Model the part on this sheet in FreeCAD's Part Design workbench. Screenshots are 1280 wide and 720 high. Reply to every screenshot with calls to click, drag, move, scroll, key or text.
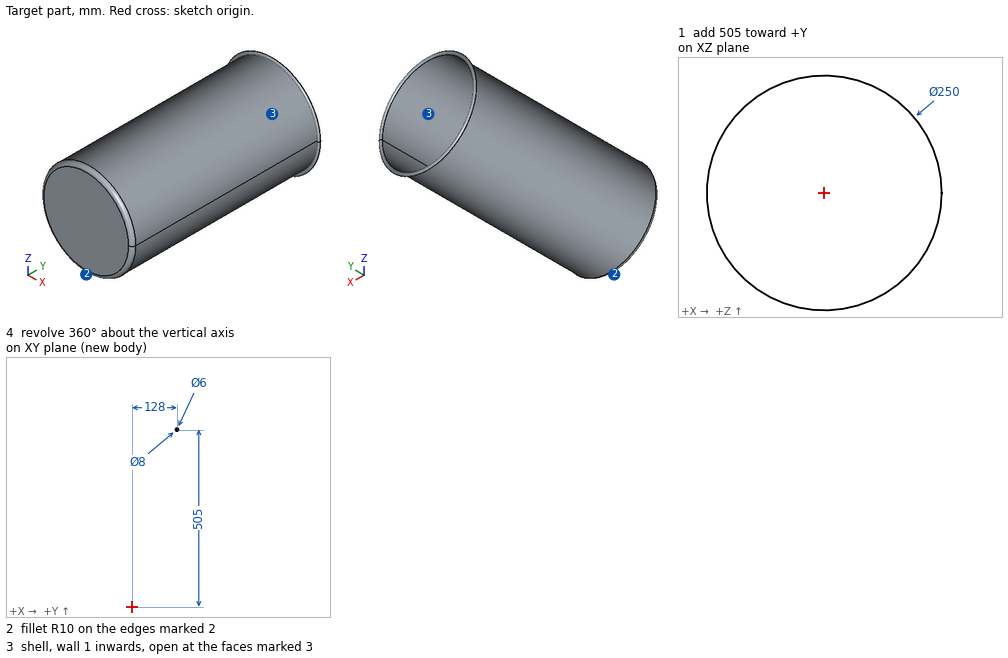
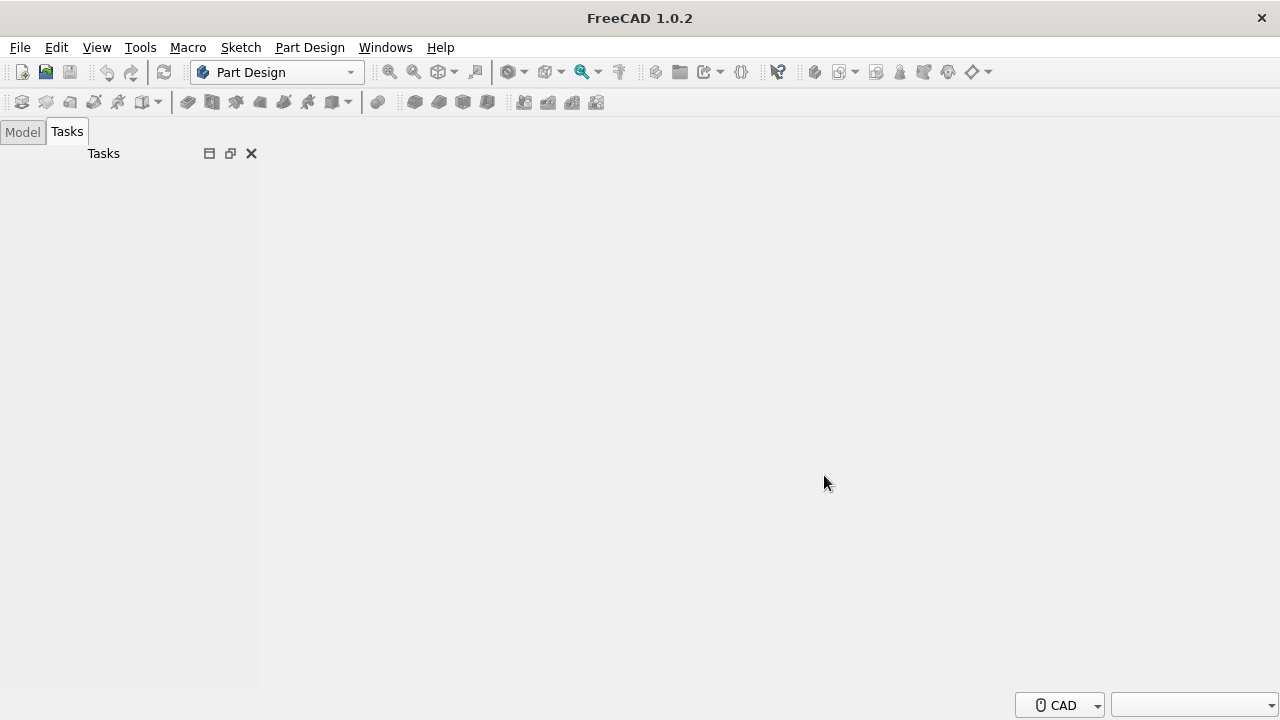
click(22, 72)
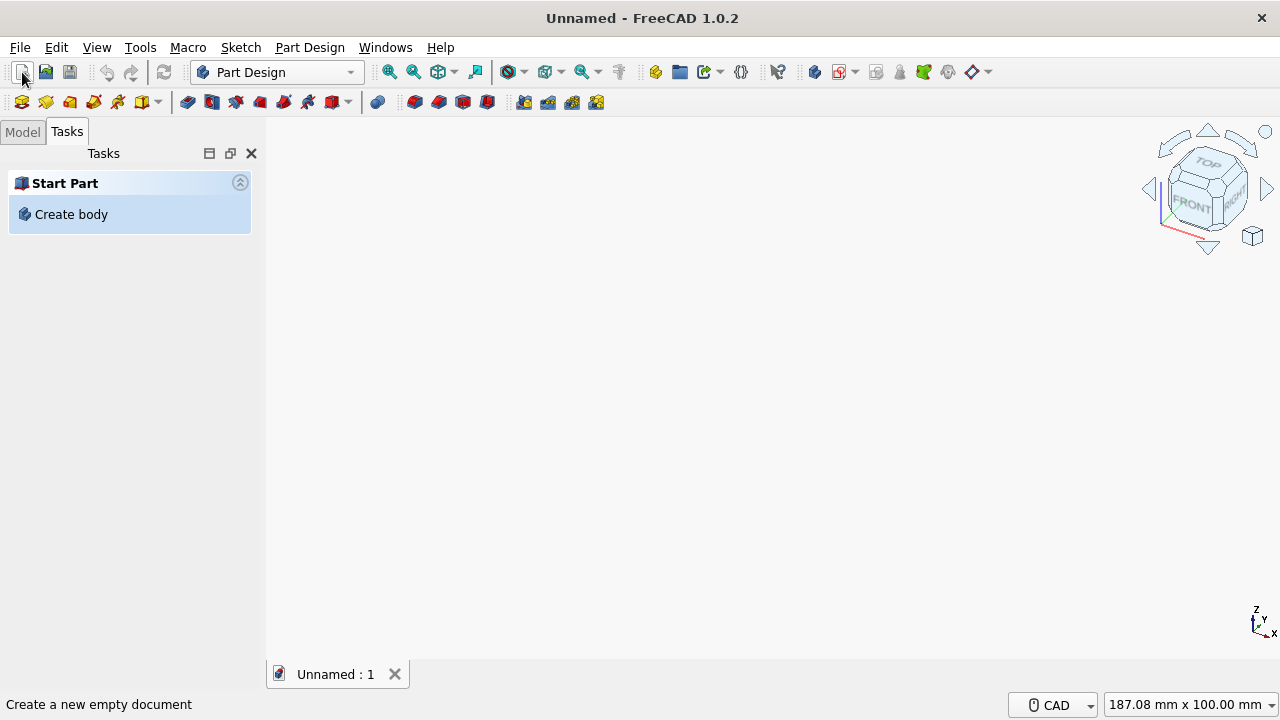
click(840, 72)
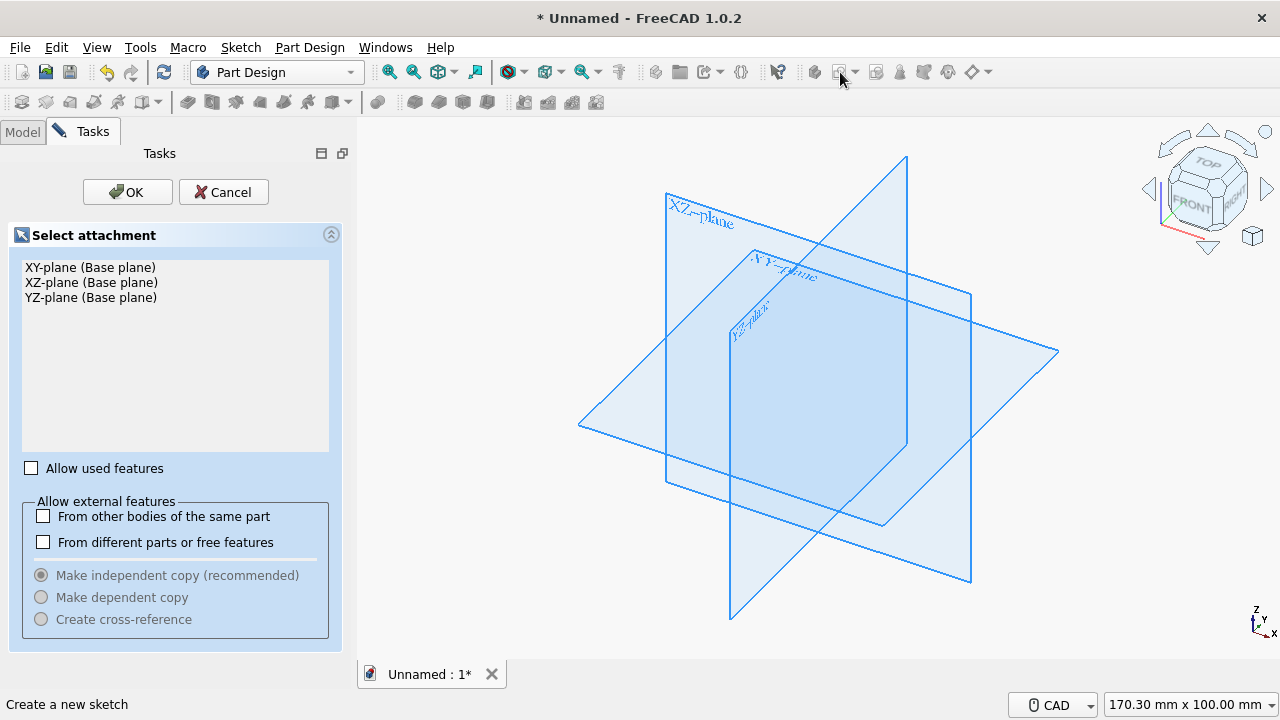
click(82, 282)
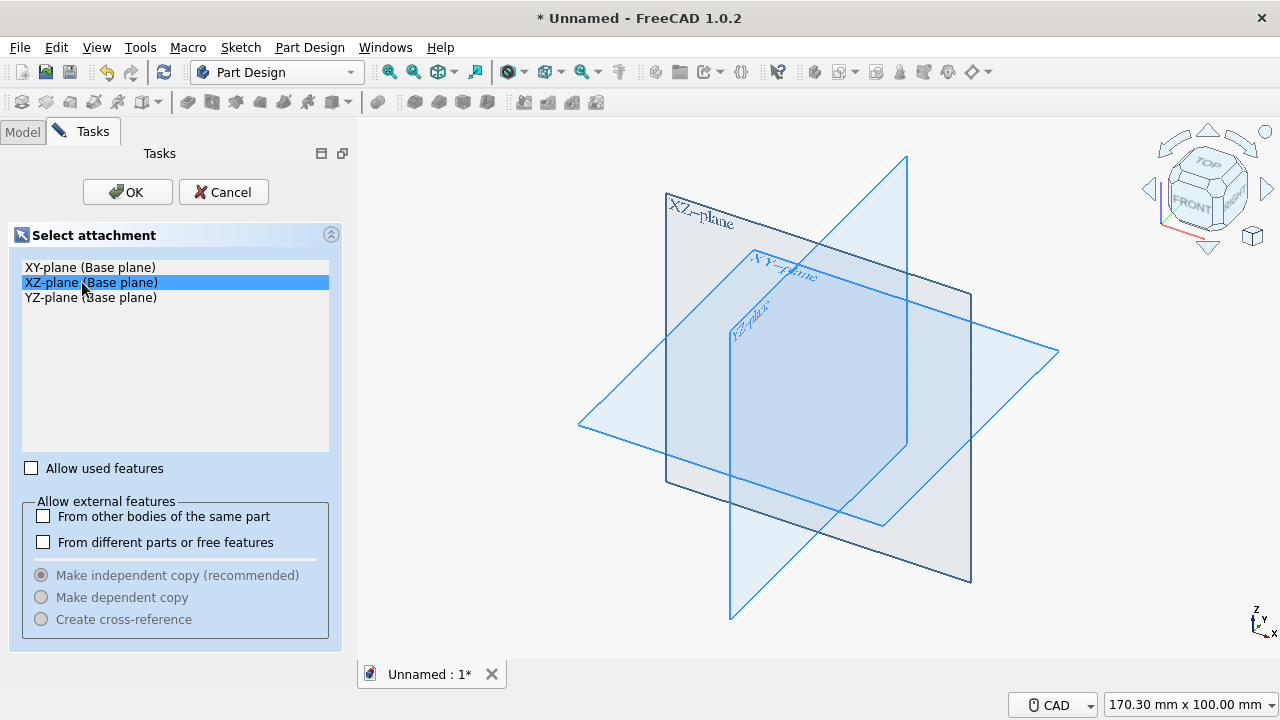
click(128, 192)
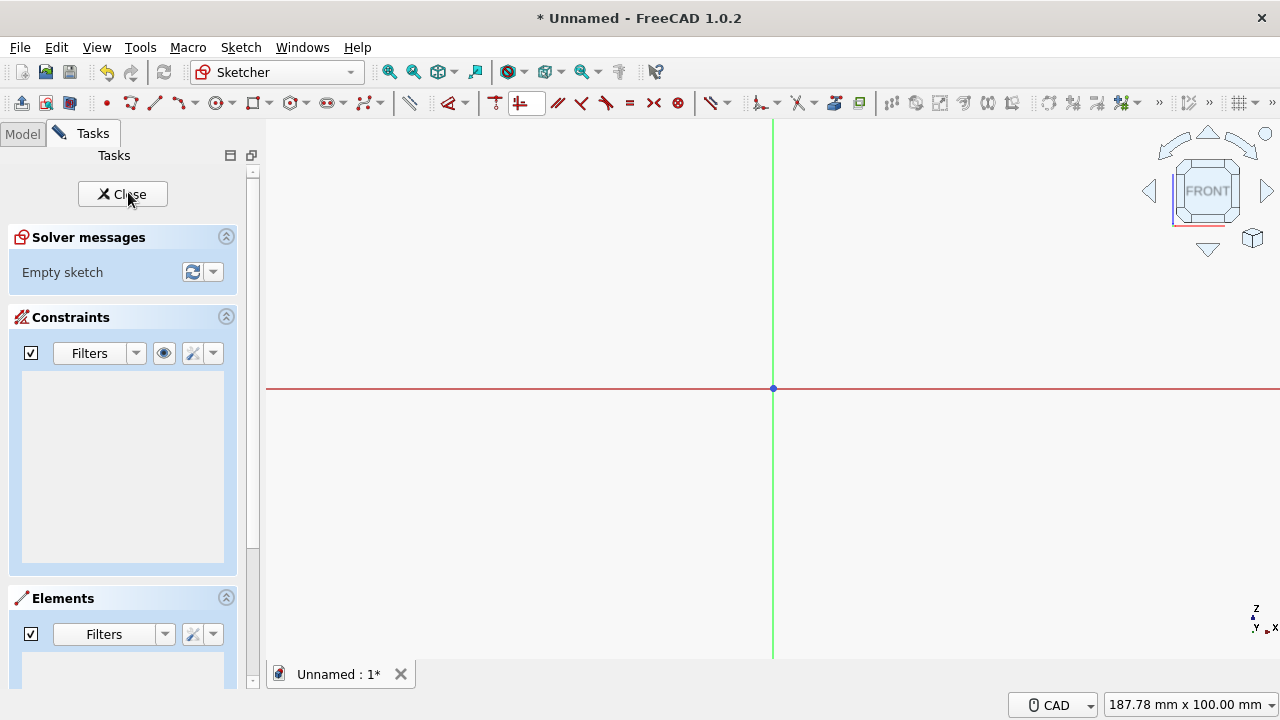
scroll(682, 389, down, 7)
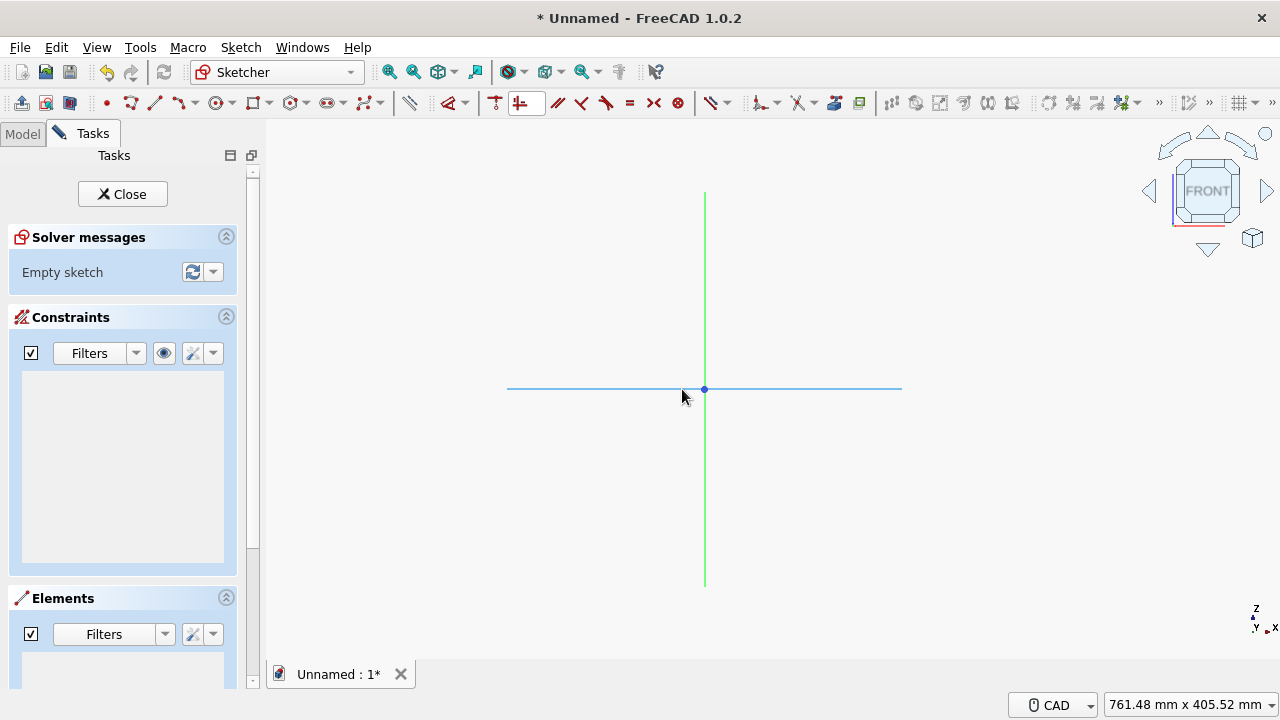
click(216, 104)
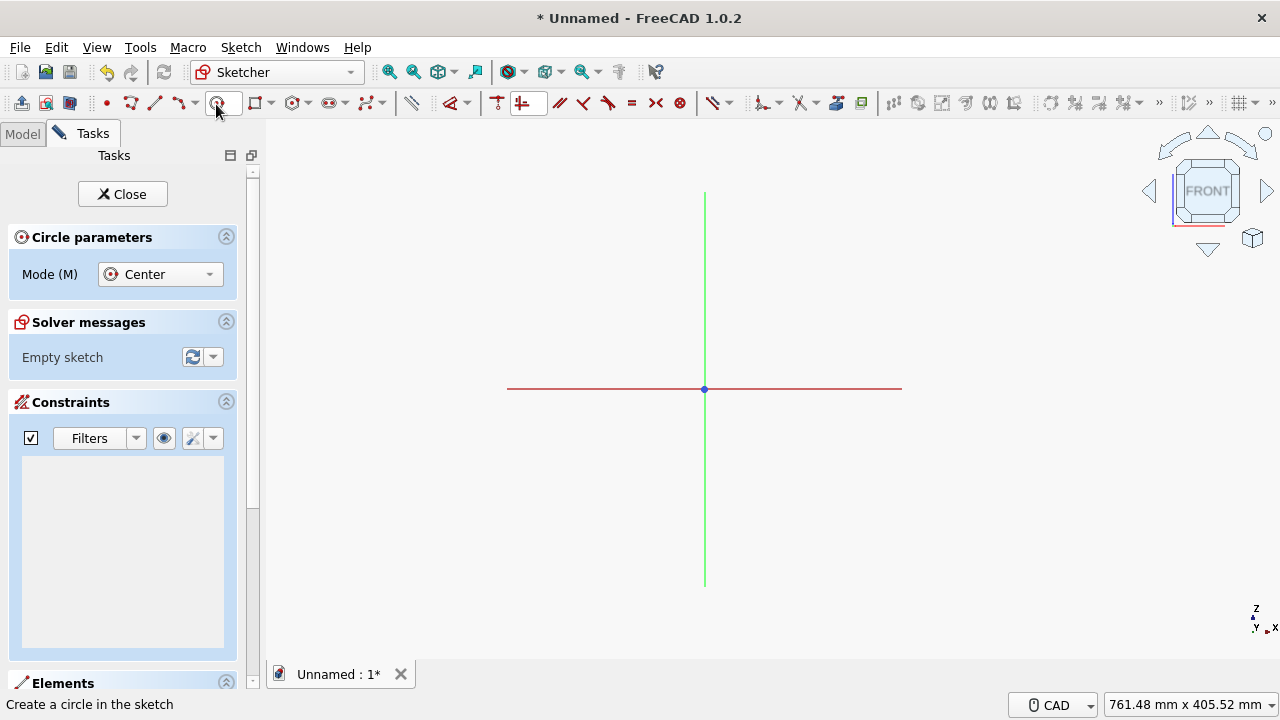
click(705, 389)
move(822, 272)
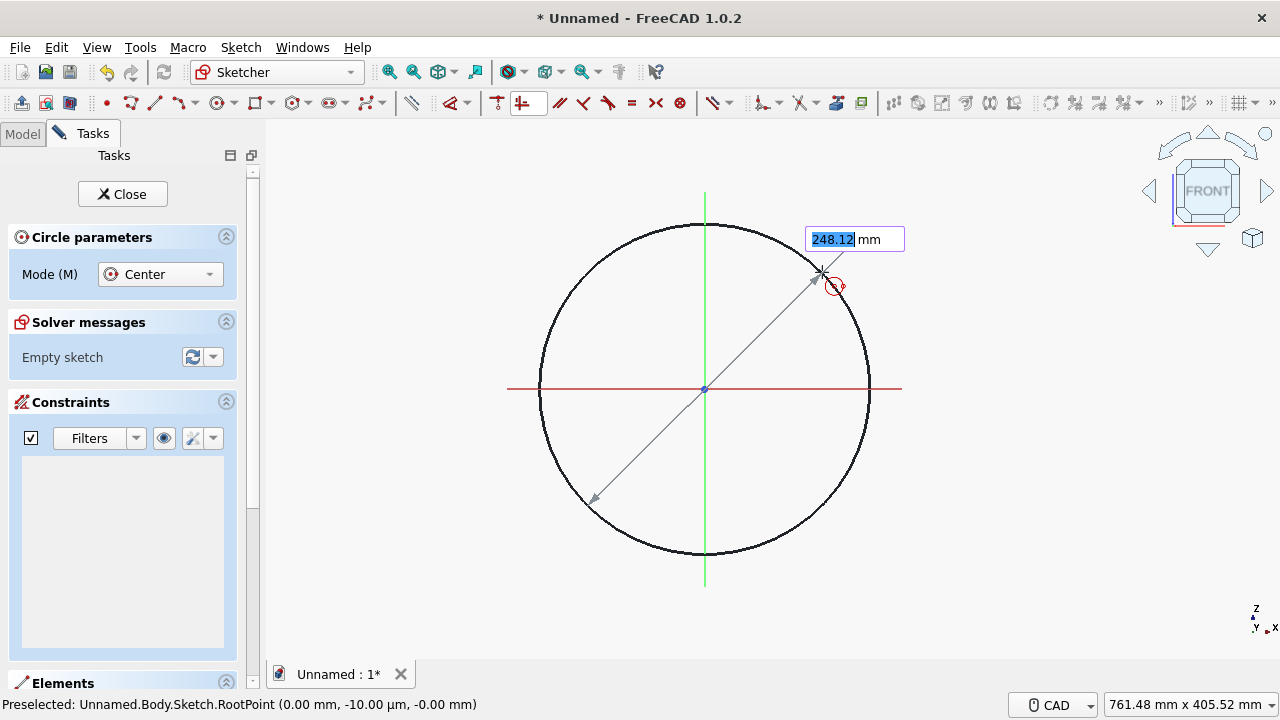
text(250)
key(Return)
key(Escape)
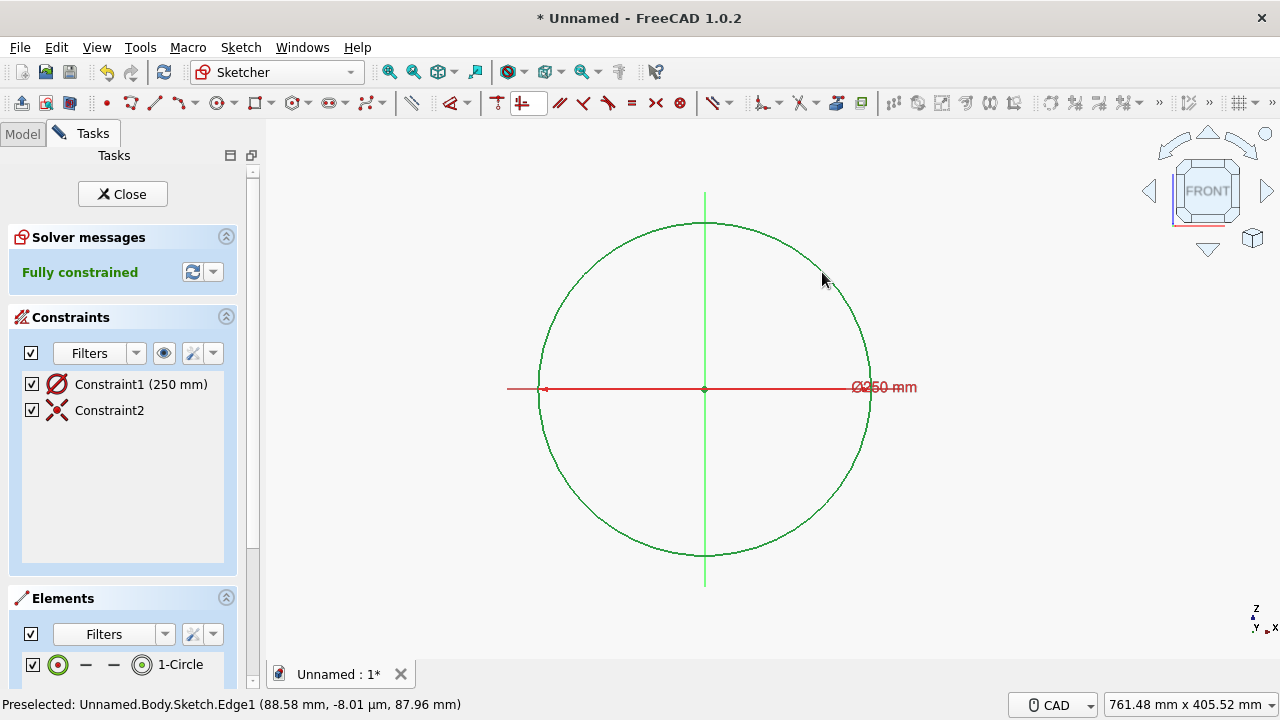
click(123, 194)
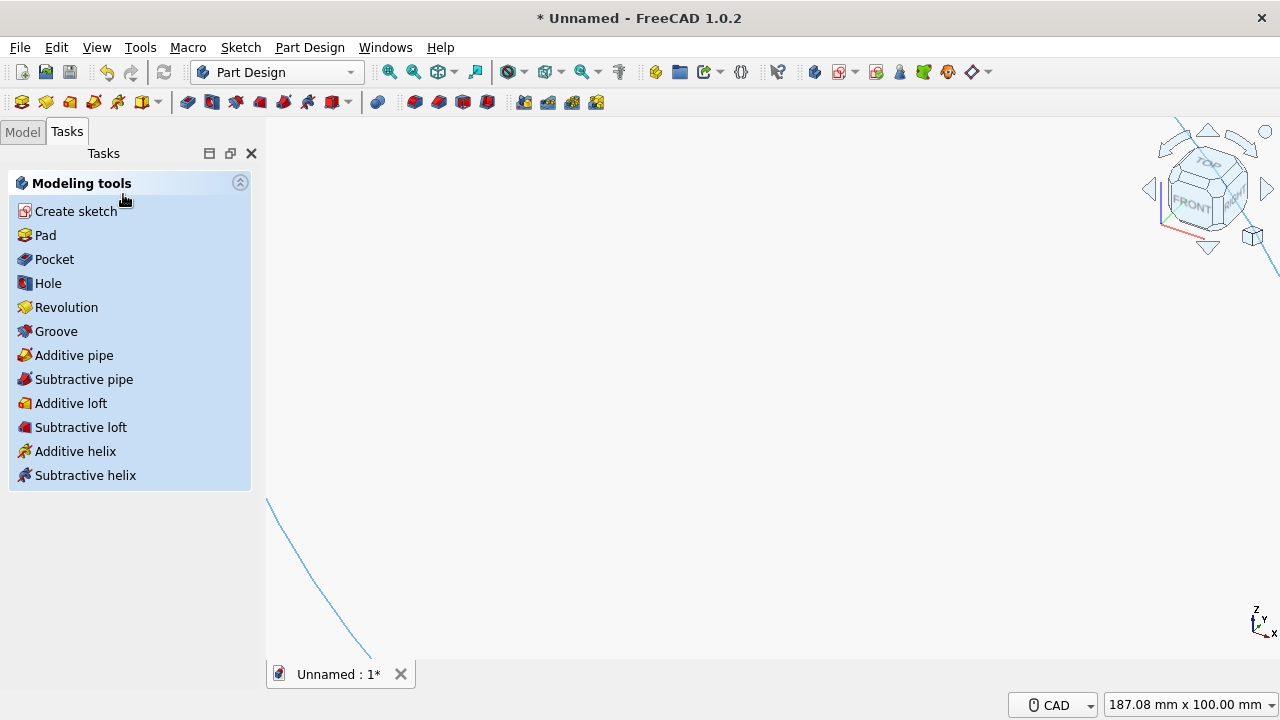
click(22, 102)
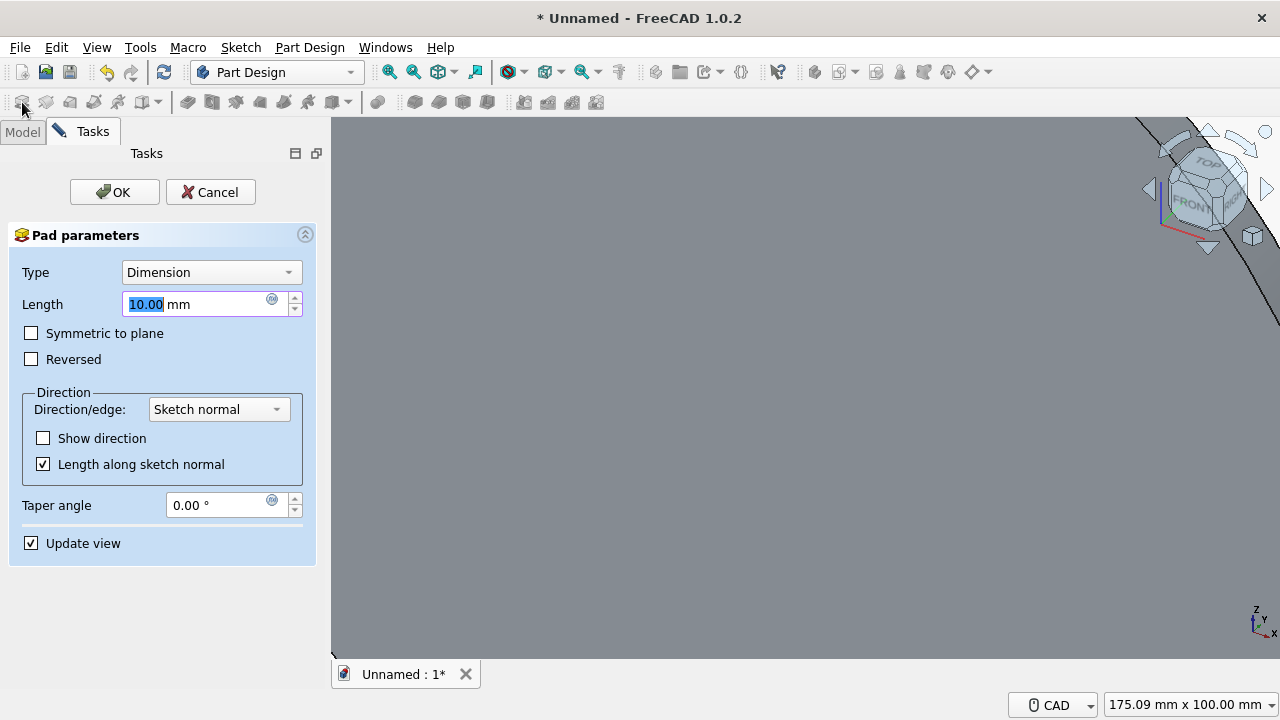
text(505)
key(Tab)